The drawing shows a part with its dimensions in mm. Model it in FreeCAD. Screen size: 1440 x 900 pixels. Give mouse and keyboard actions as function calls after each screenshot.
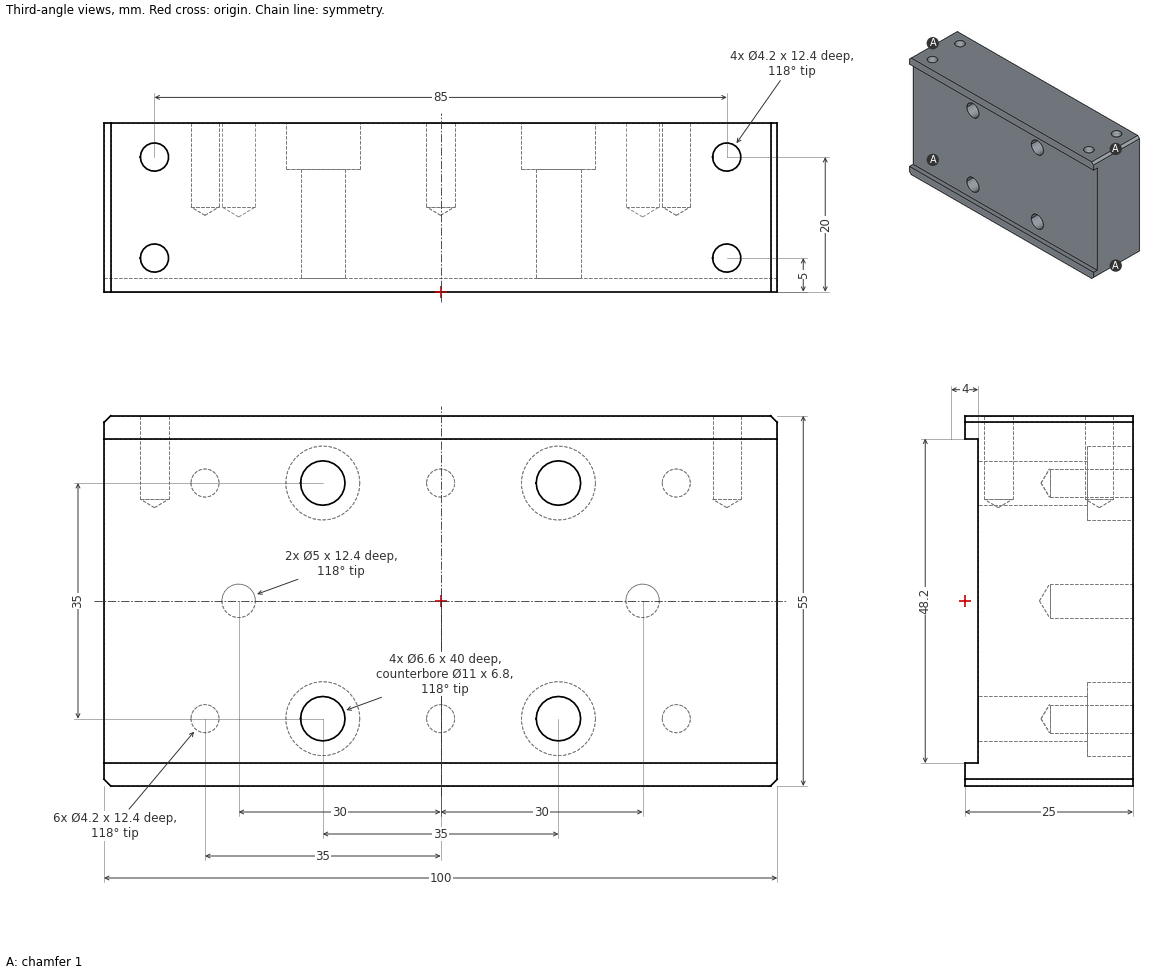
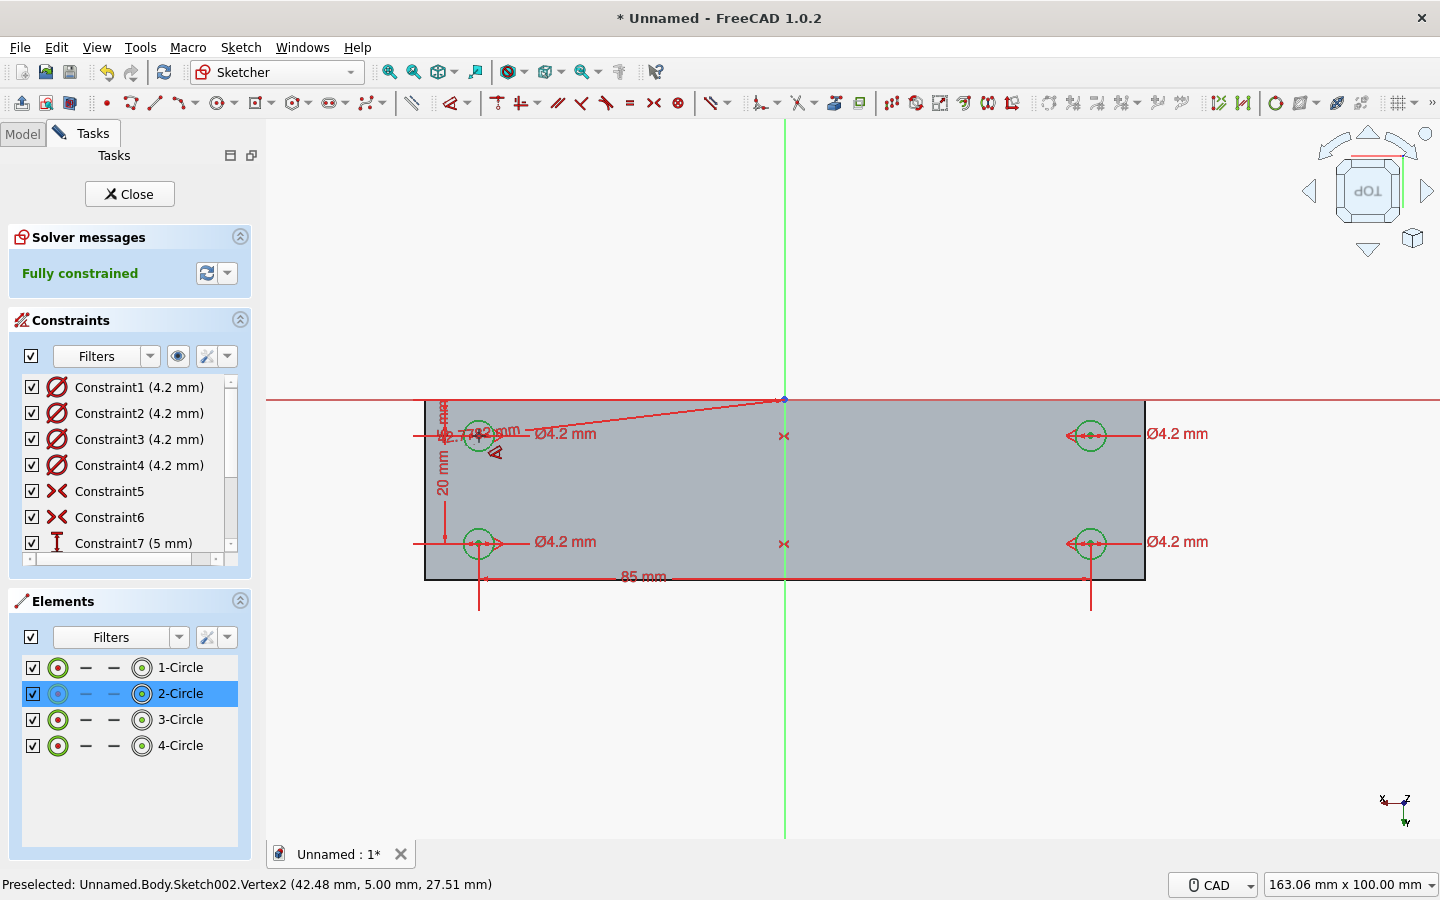
click(1091, 544)
click(926, 578)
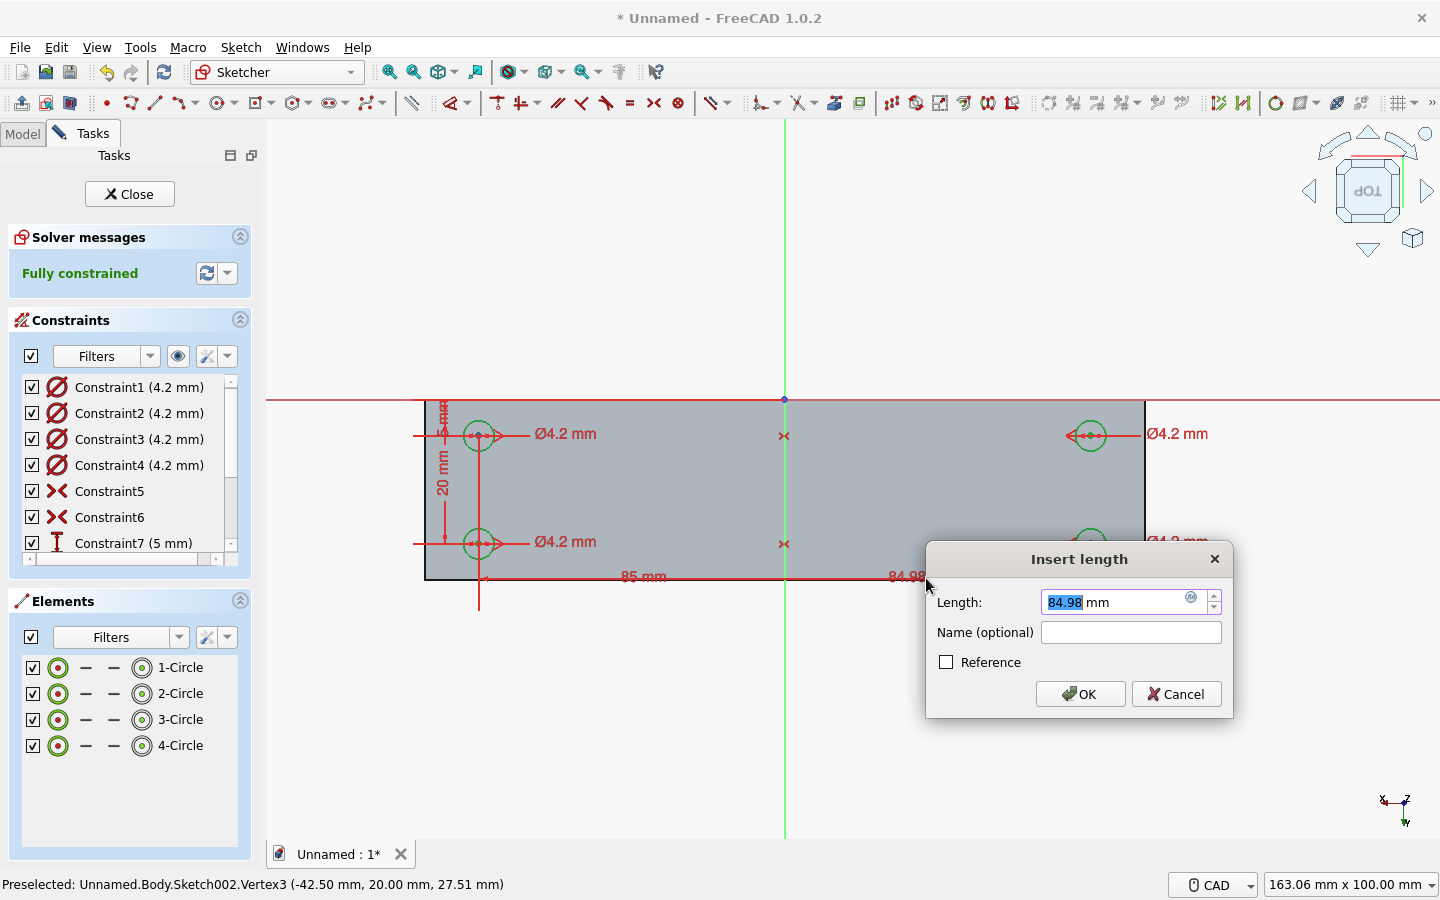
text(85)
key(Return)
key(Escape)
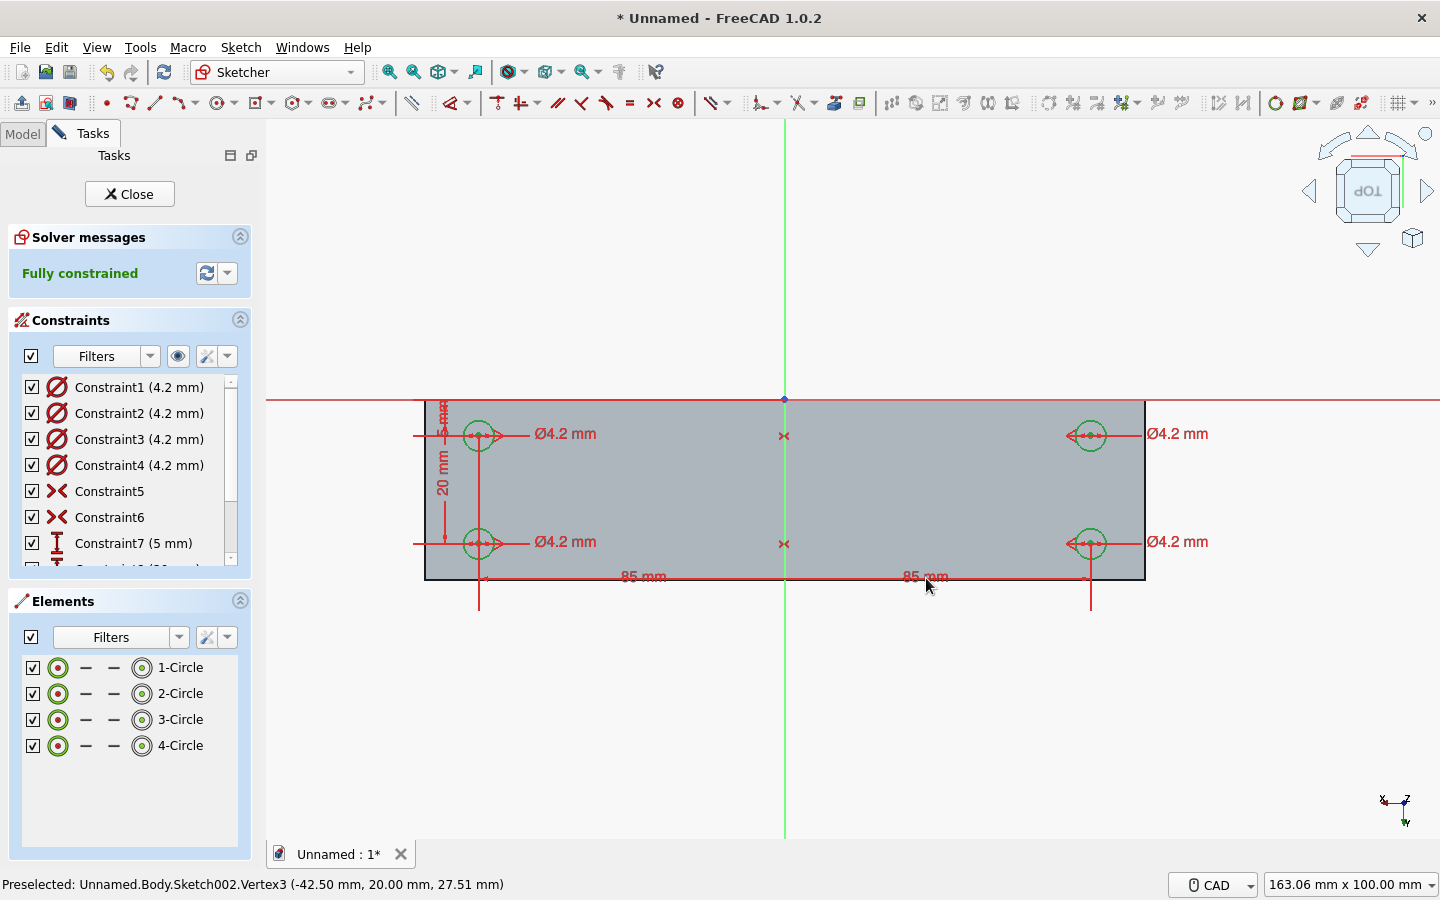
click(130, 194)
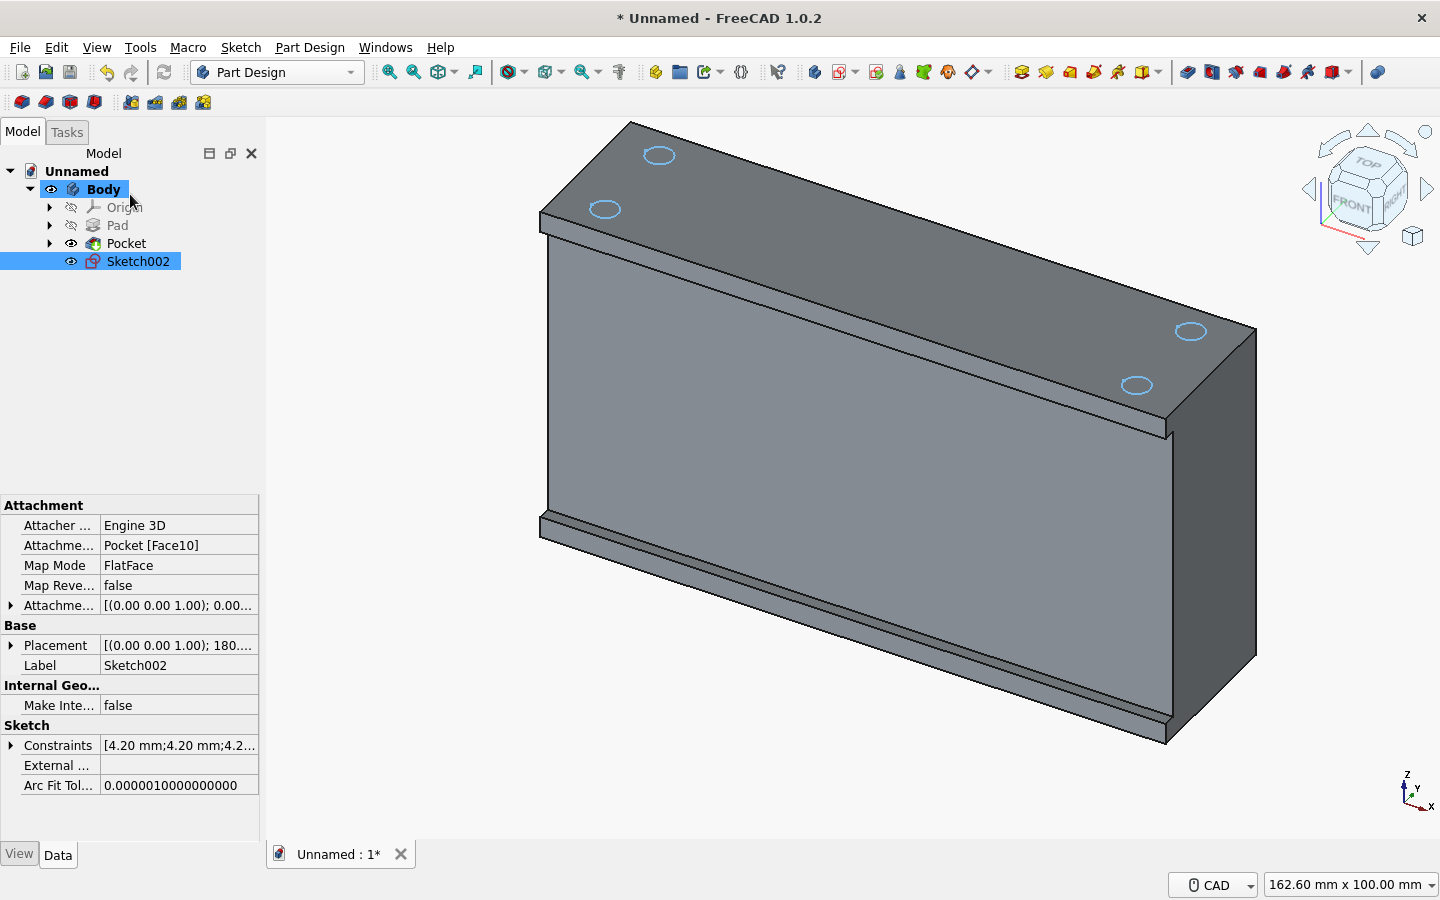
click(1212, 72)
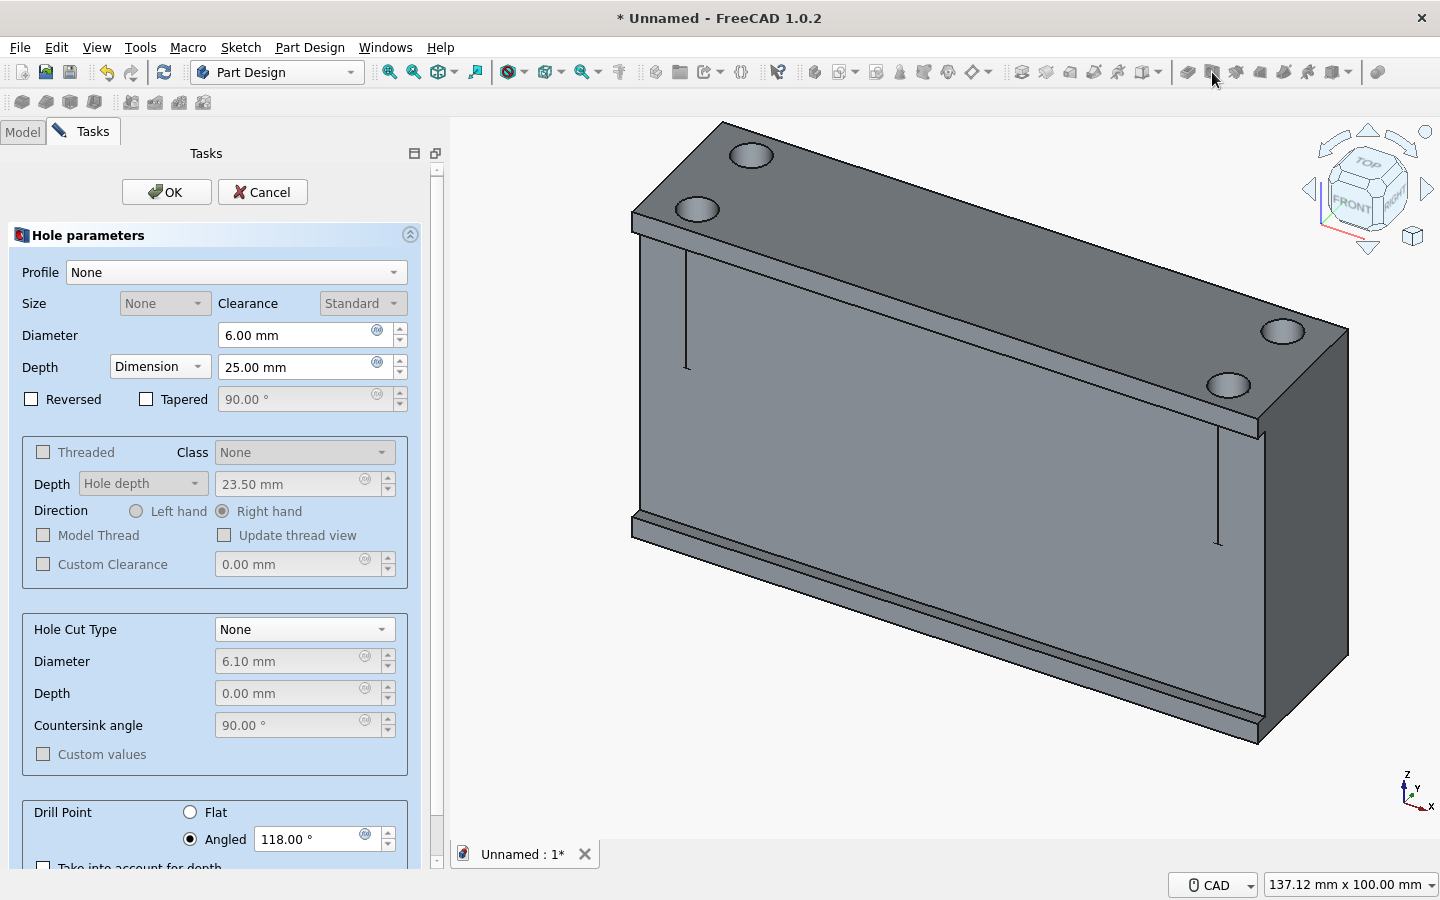
triple_click(305, 335)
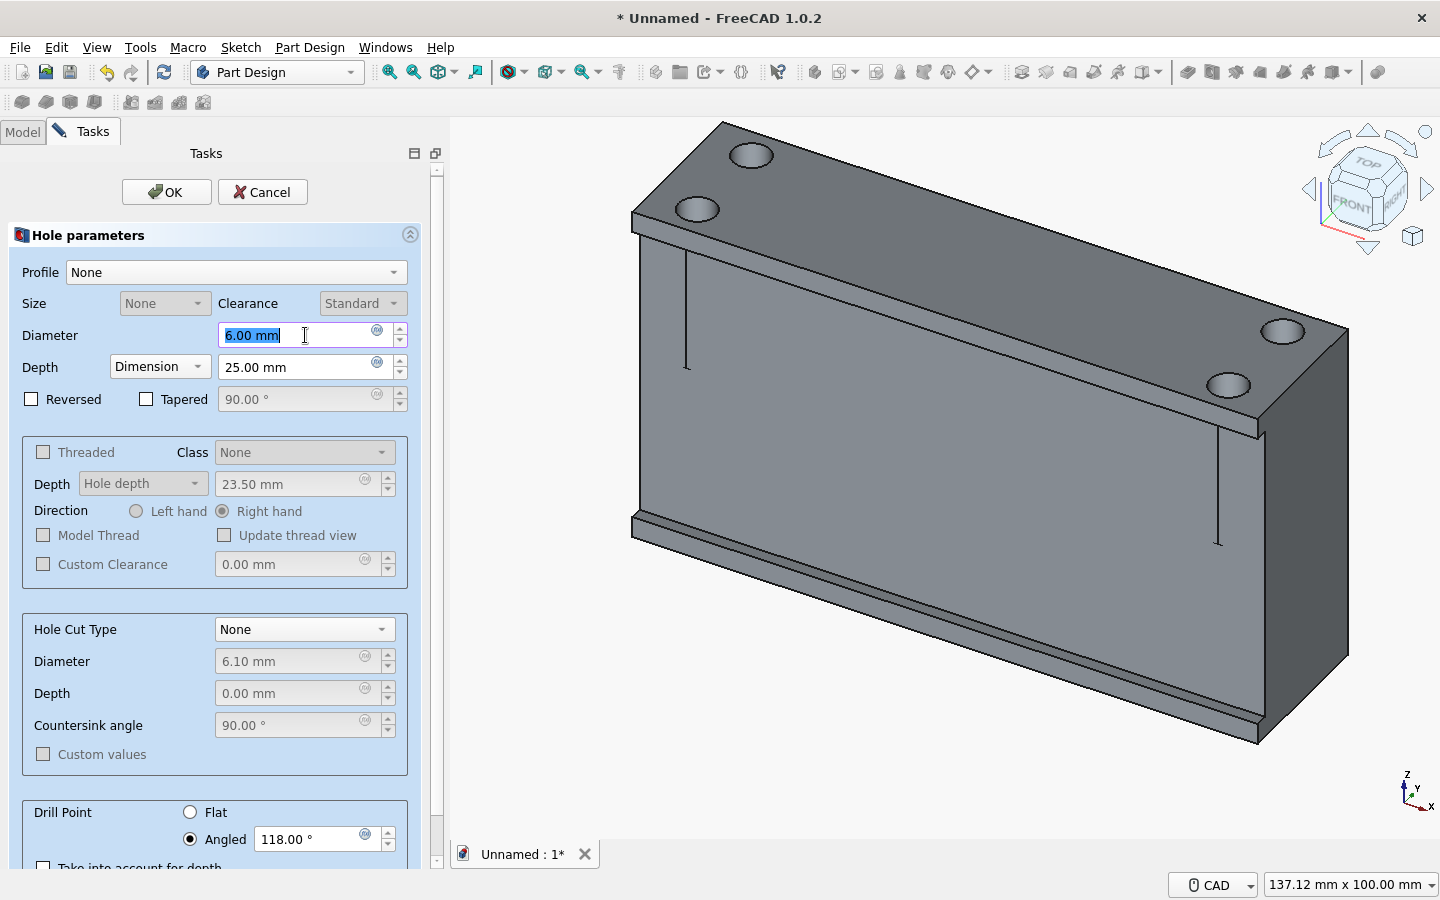
text(4.2)
key(Tab)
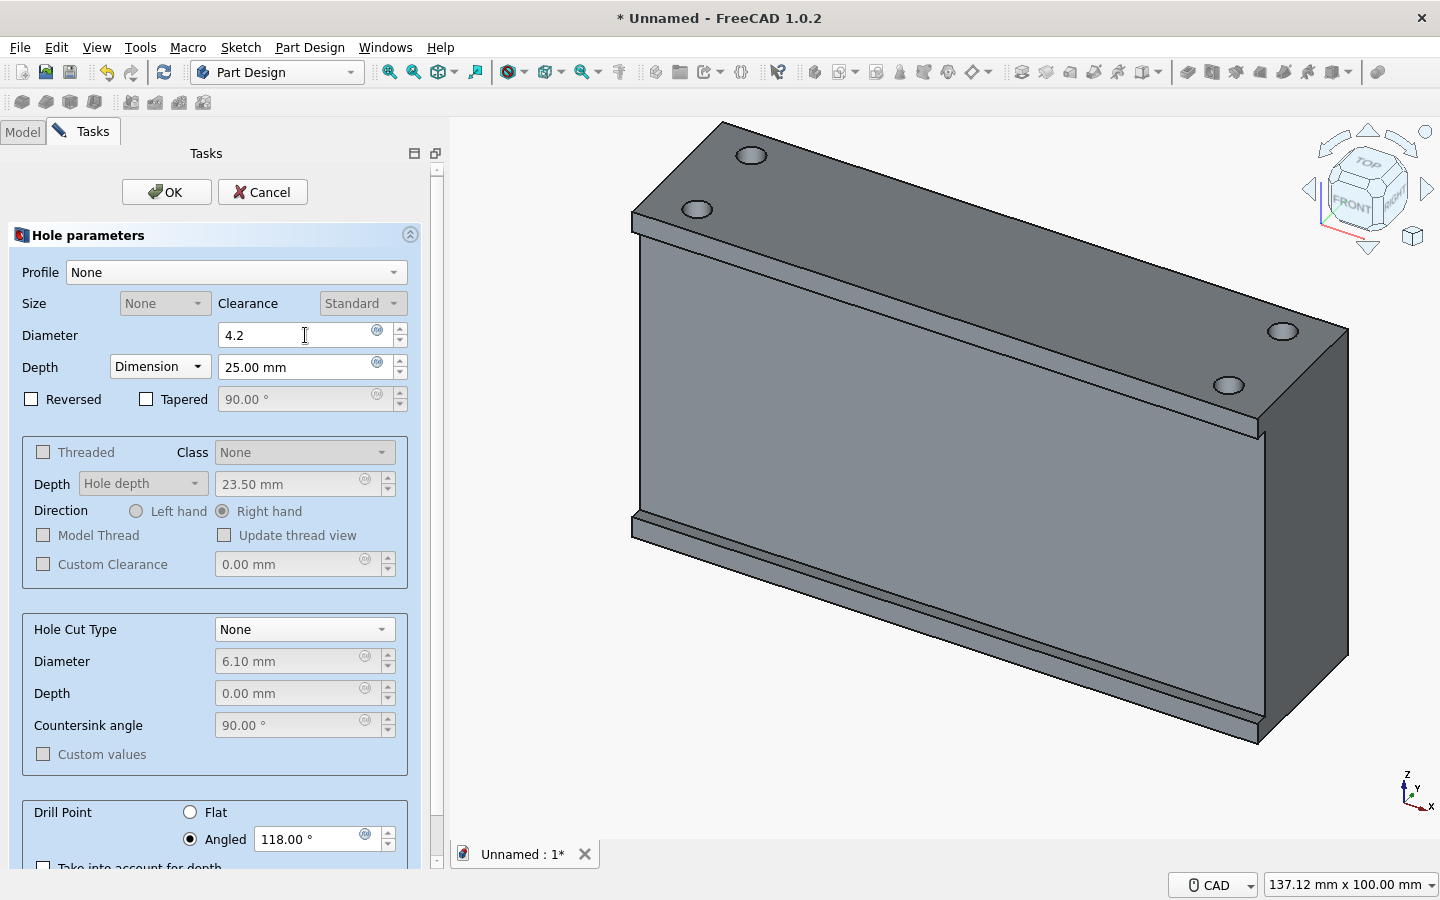
triple_click(305, 367)